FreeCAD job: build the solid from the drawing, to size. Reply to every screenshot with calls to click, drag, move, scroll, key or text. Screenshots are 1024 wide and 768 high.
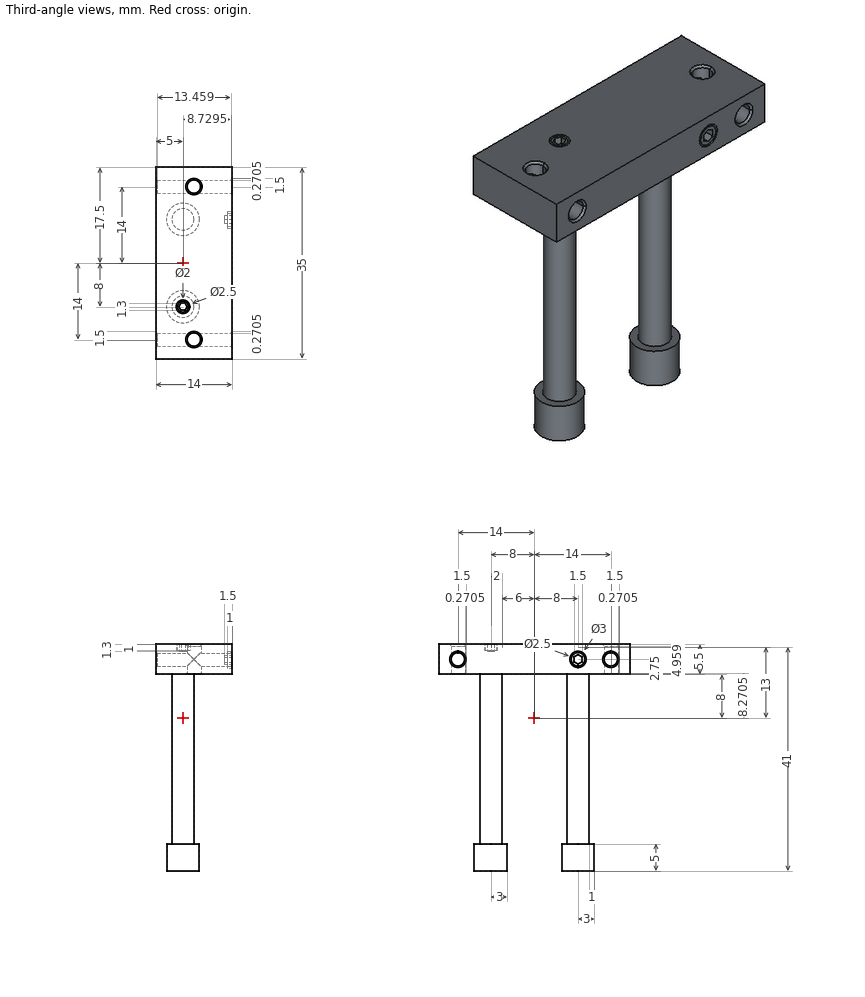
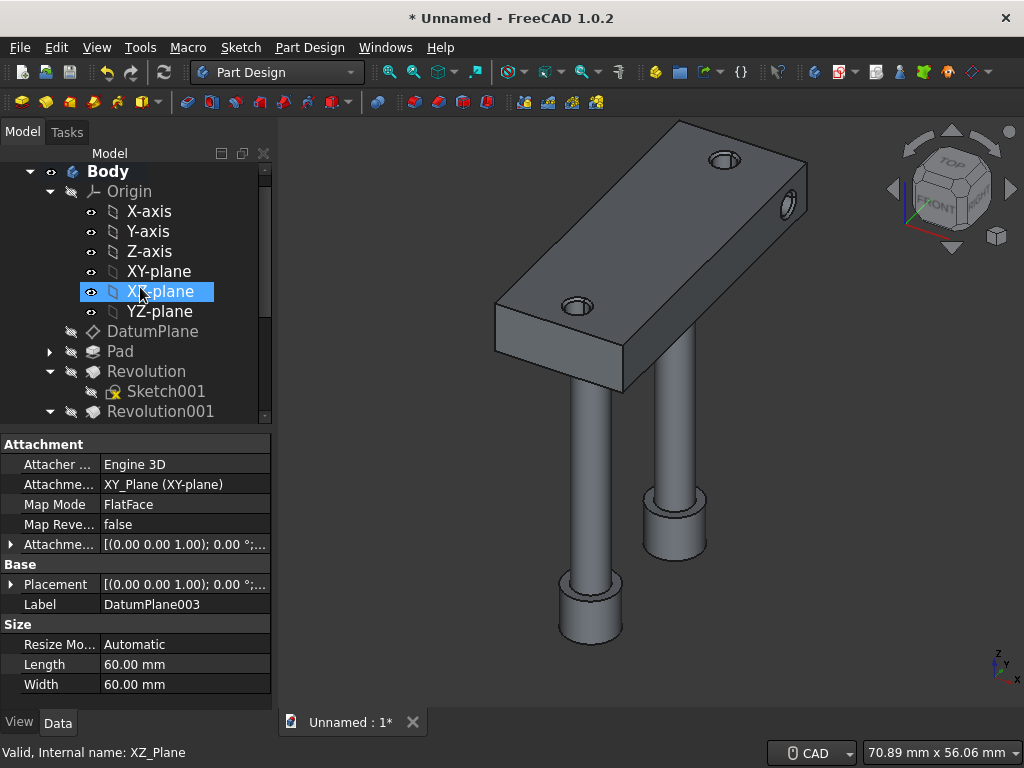
click(136, 292)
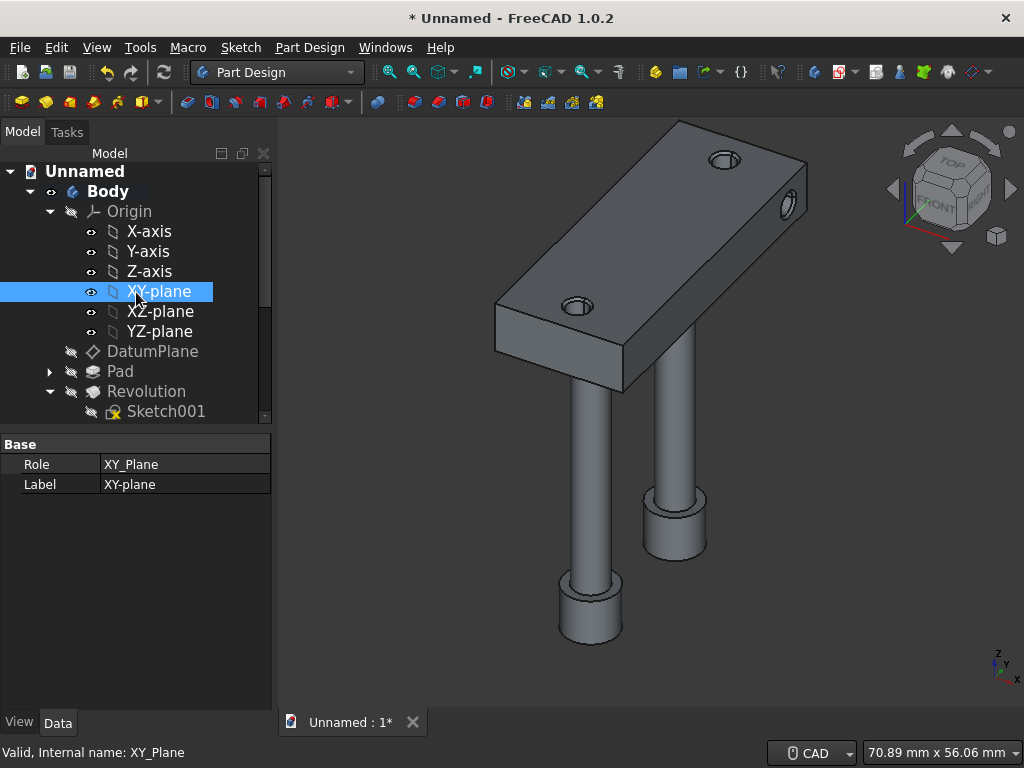
click(972, 72)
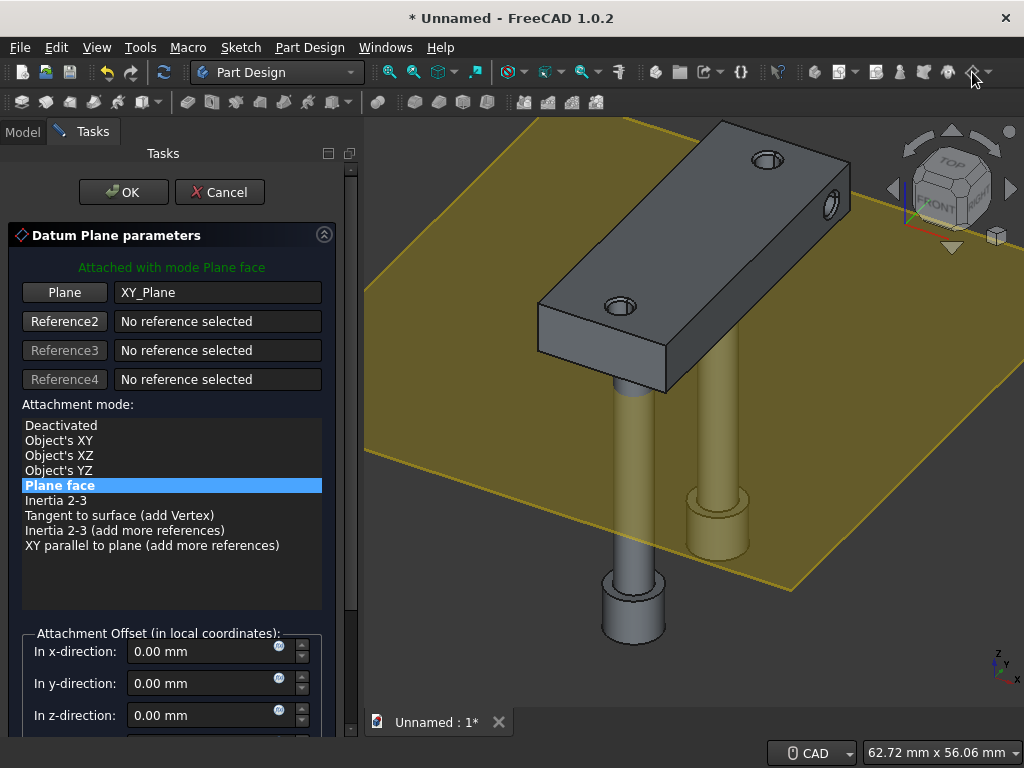
triple_click(210, 715)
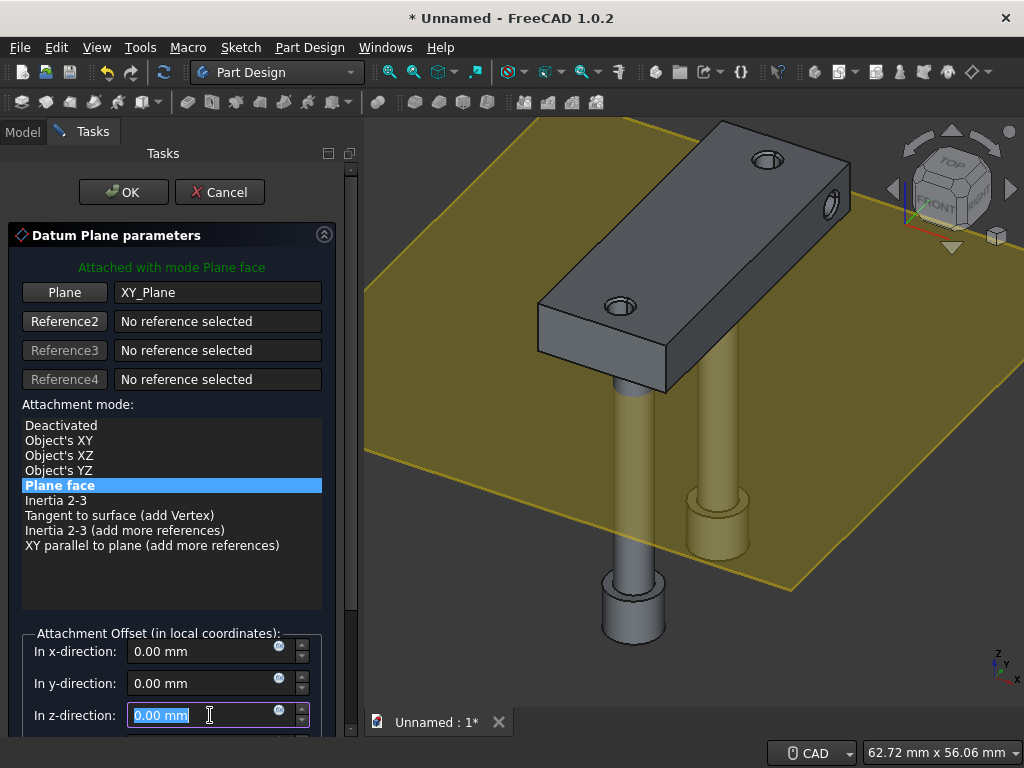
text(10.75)
key(Tab)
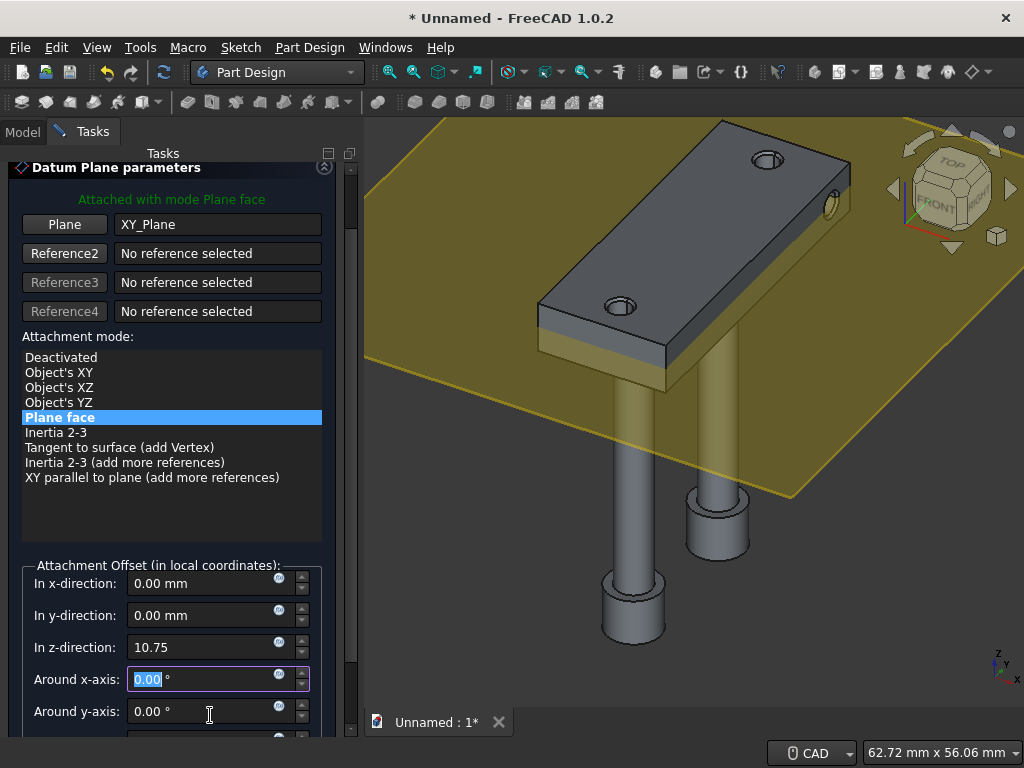
scroll(351, 450, up, 2)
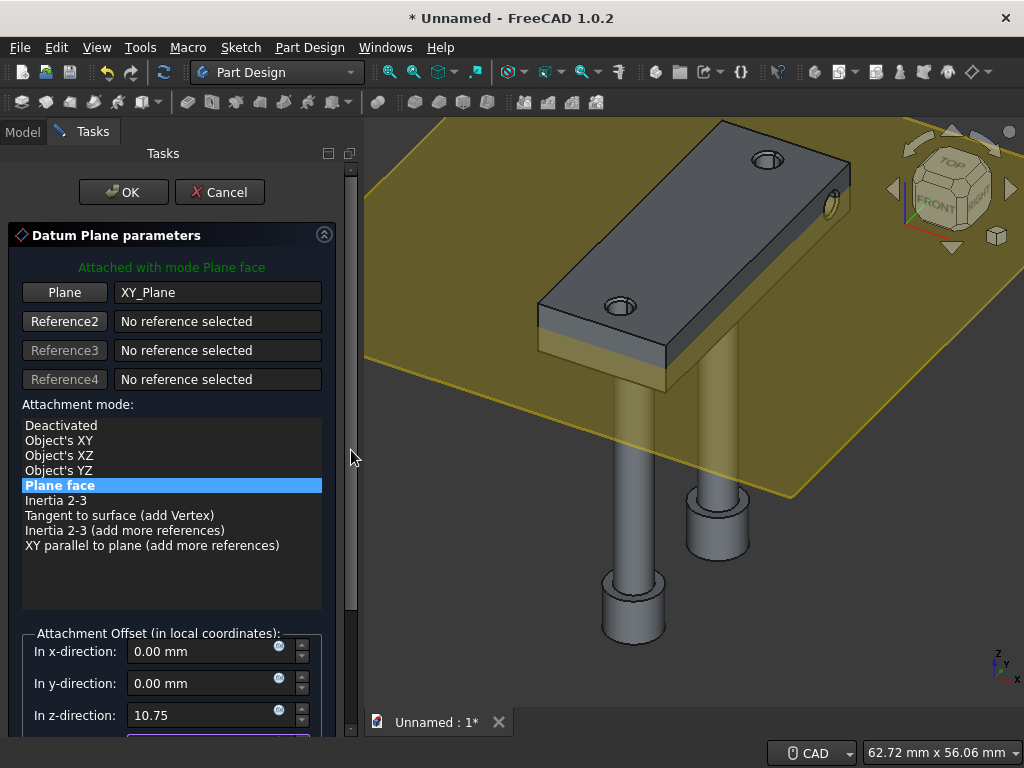
click(124, 192)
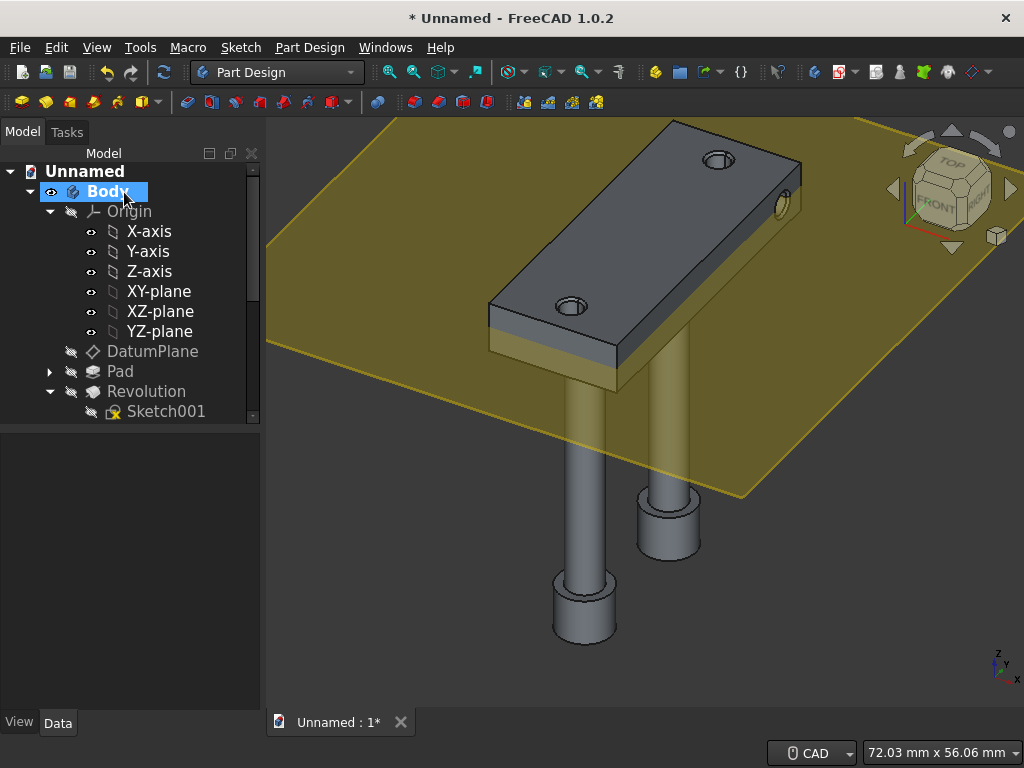
scroll(100, 287, down, 3)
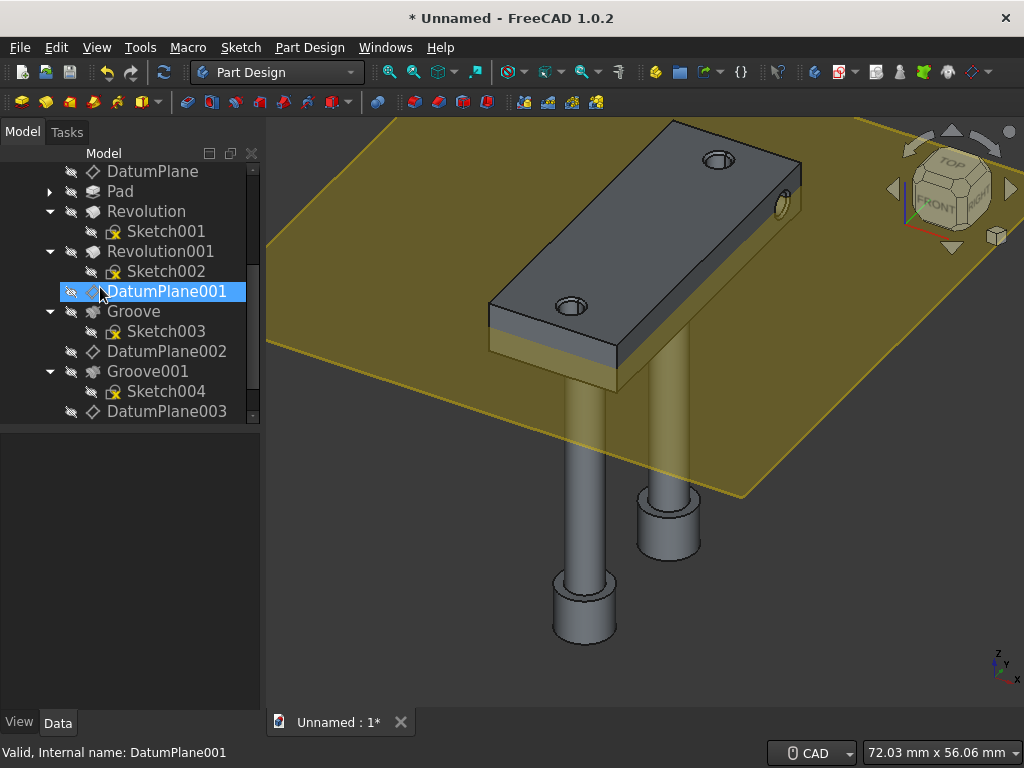
scroll(140, 287, up, 15)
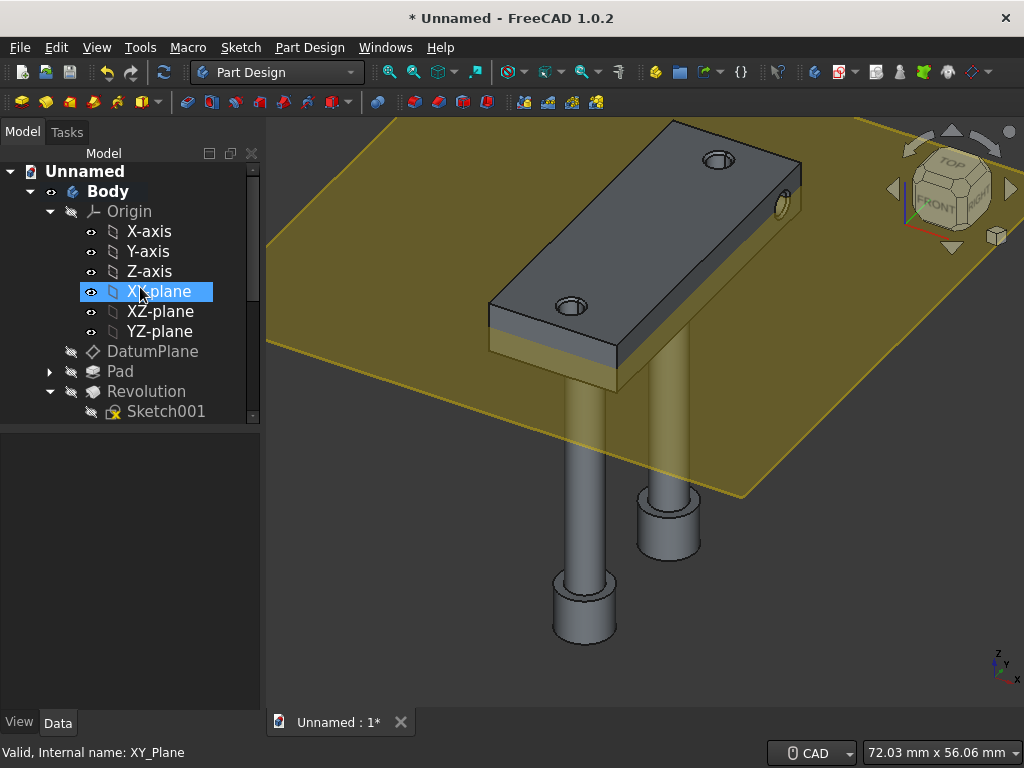
scroll(100, 287, down, 6)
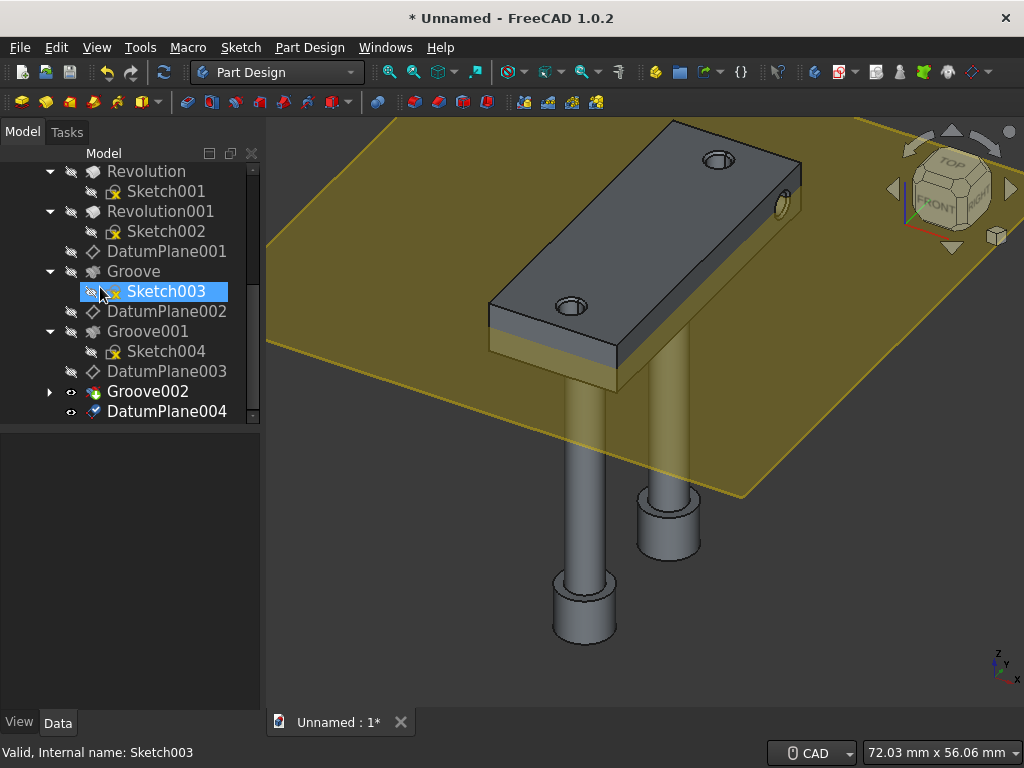
click(116, 412)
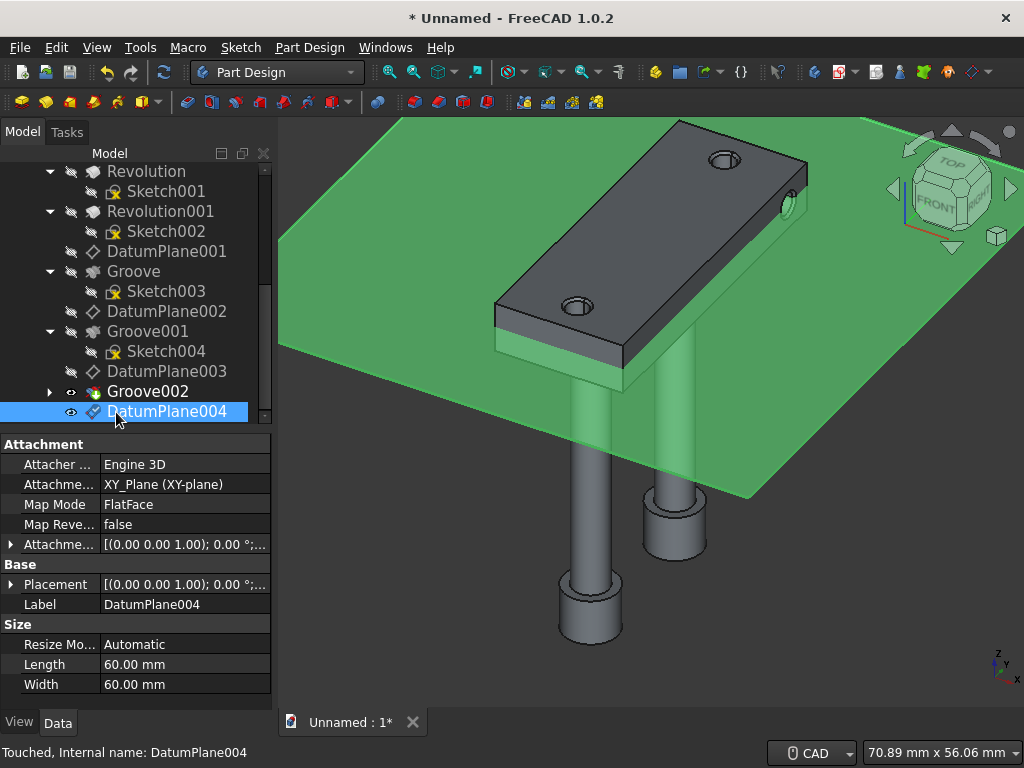
click(840, 72)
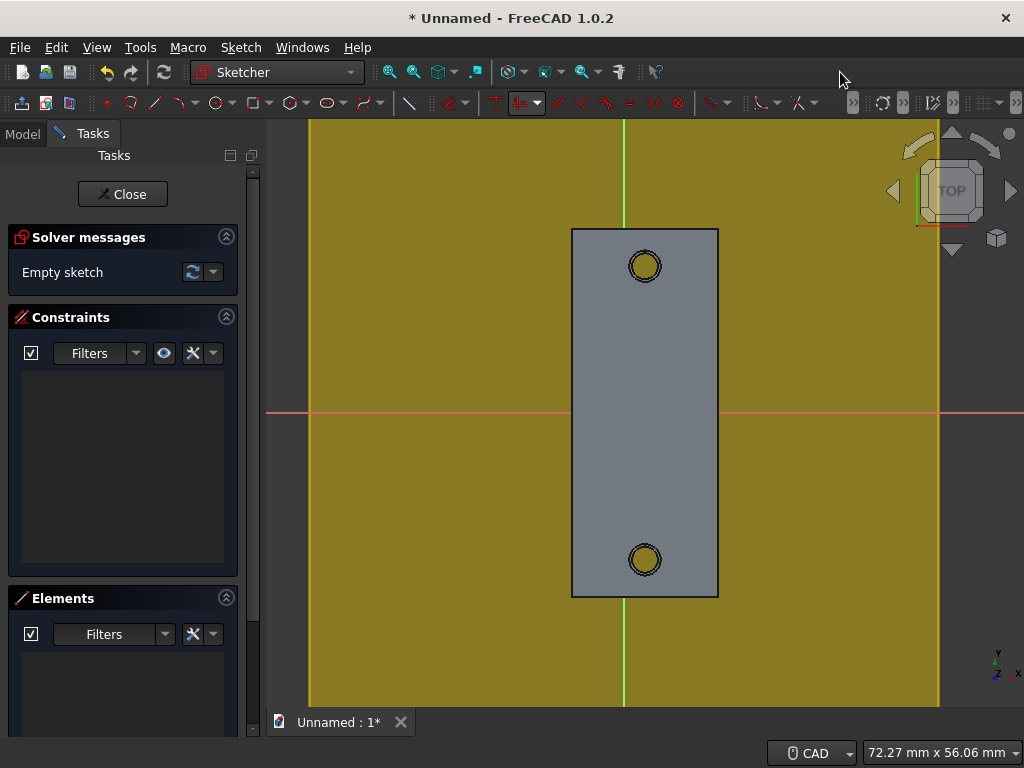
click(70, 104)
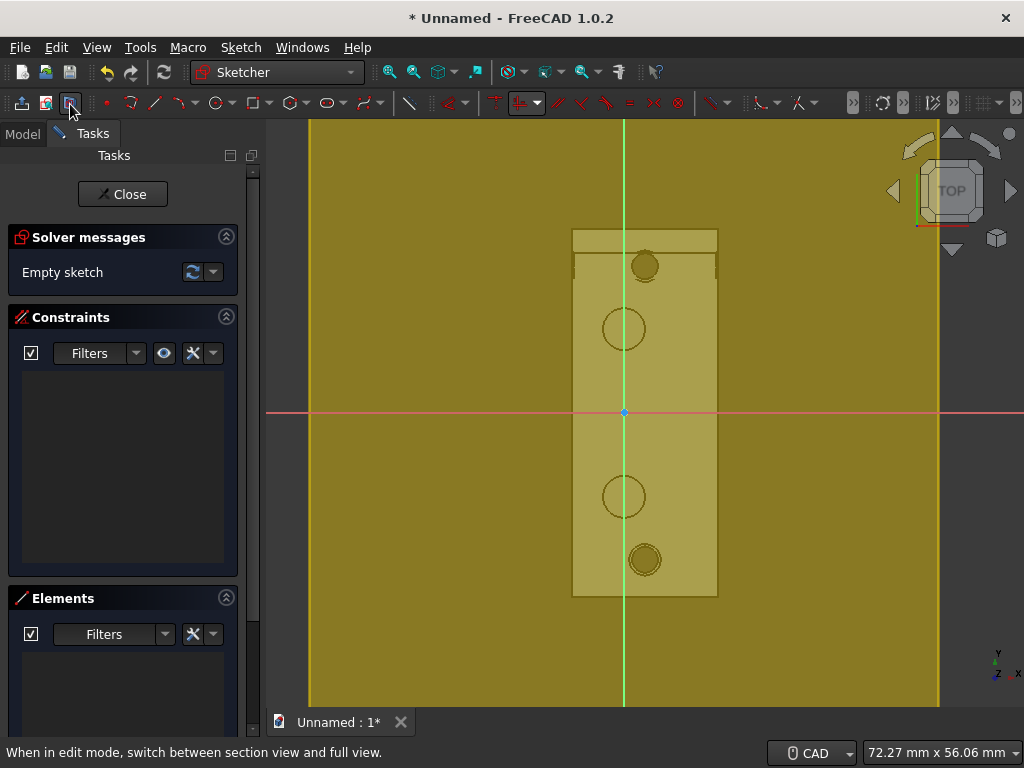
scroll(663, 576, up, 3)